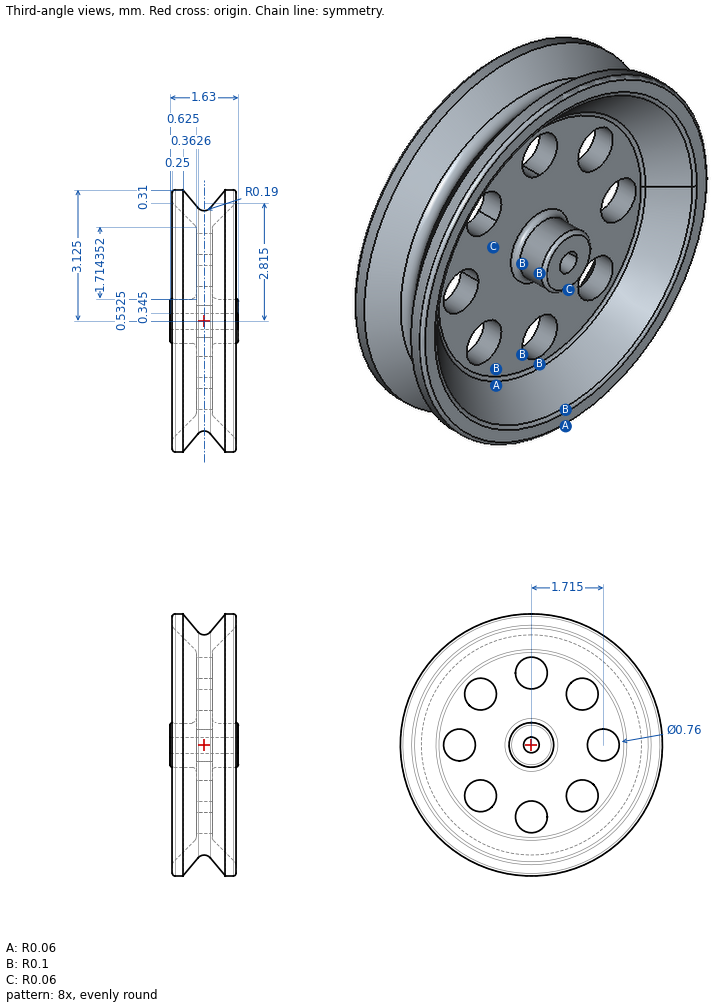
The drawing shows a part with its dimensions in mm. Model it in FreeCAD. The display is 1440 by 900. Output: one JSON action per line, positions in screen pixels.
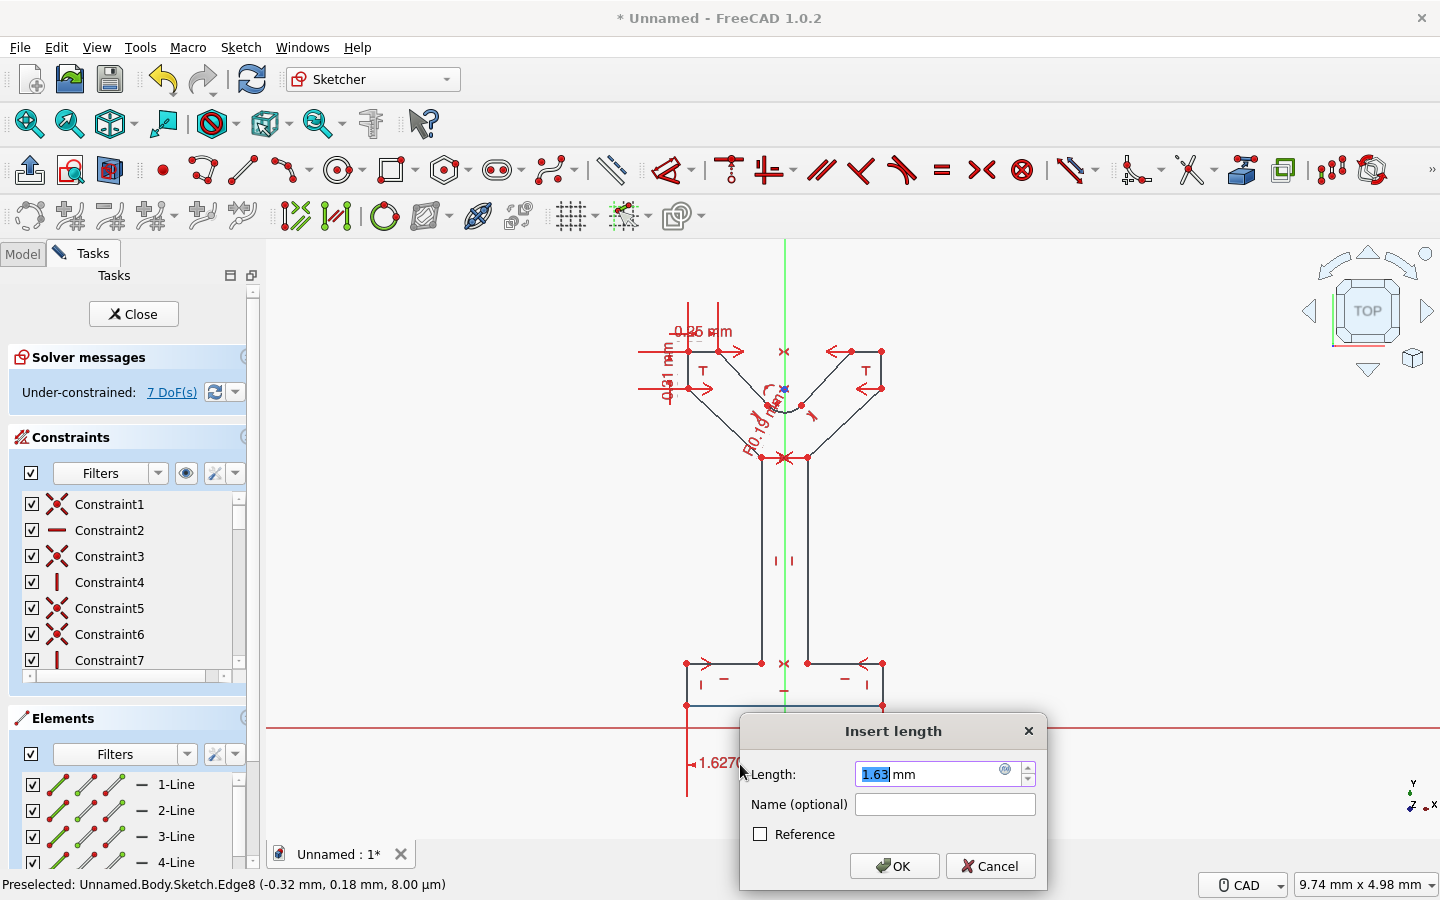
{"action": "type", "text": "1.63"}
{"action": "key", "text": "Return"}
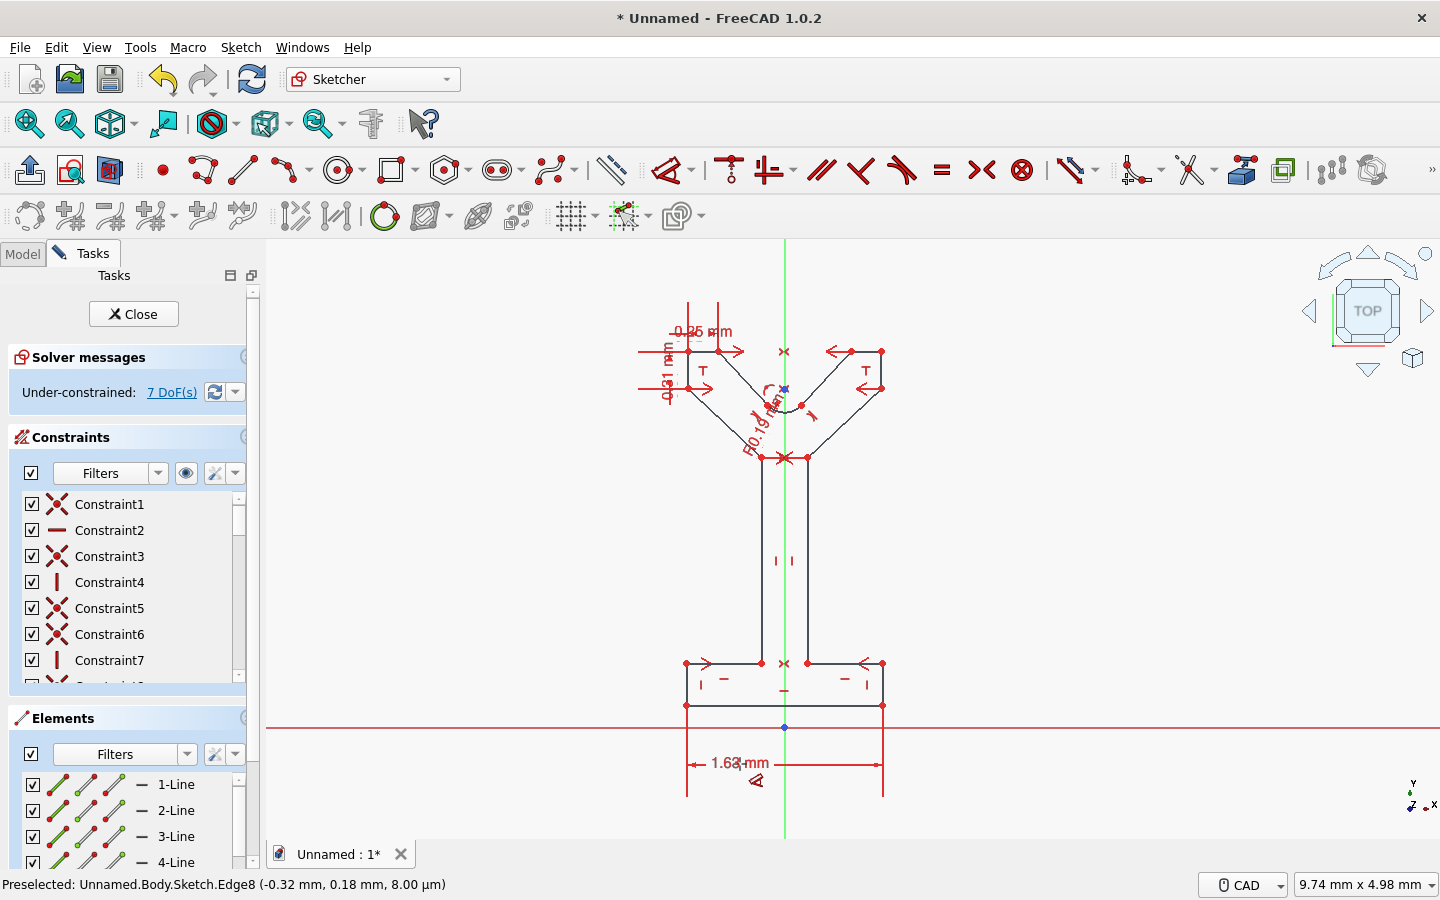
{"action": "left_click", "coordinate": [739, 664]}
{"action": "left_click", "coordinate": [724, 630]}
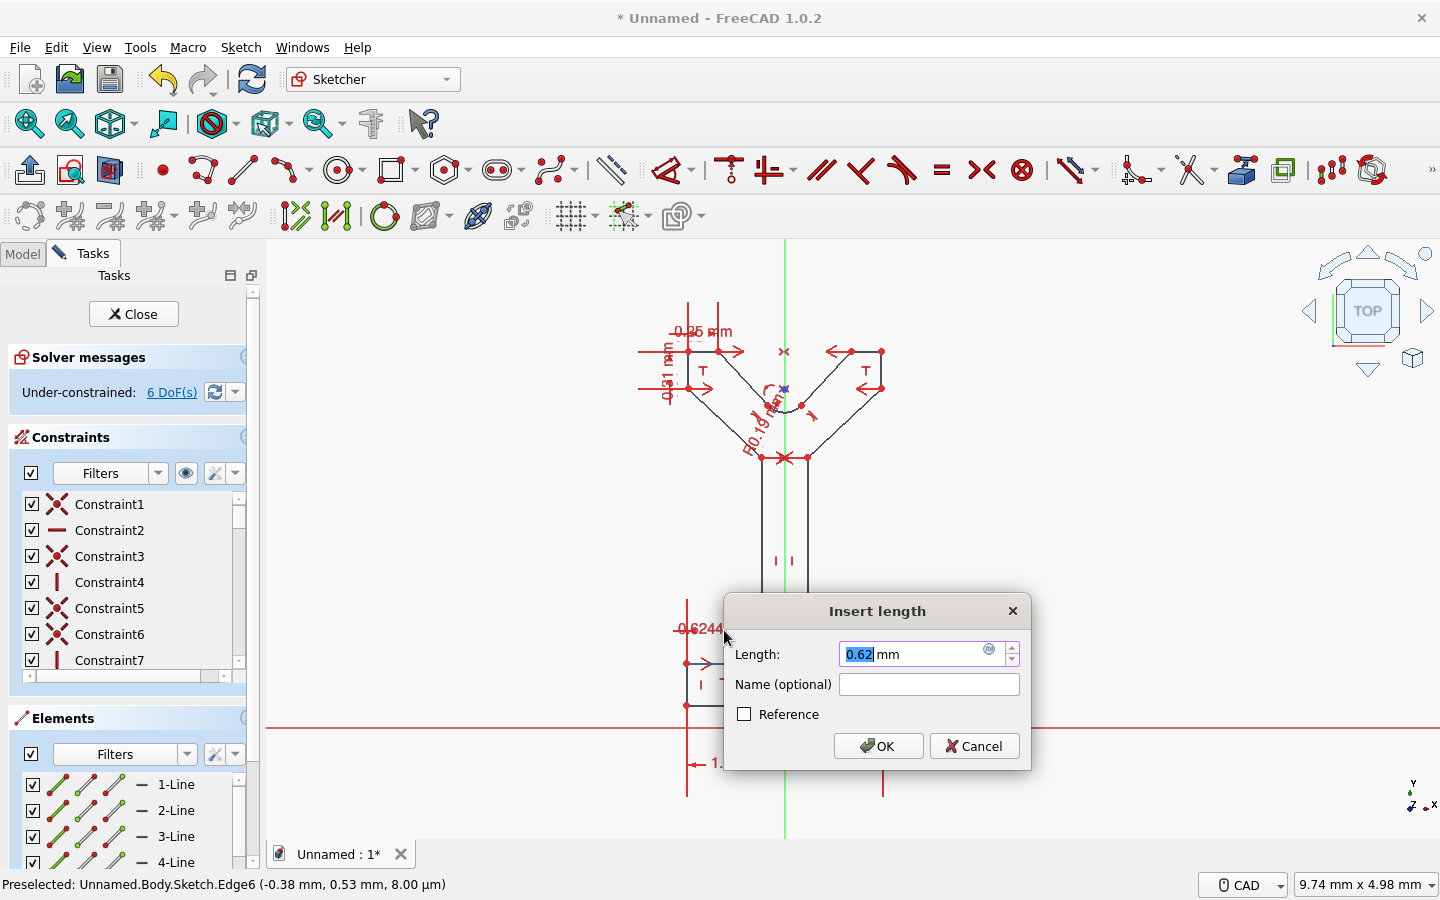
{"action": "type", "text": "0.625"}
{"action": "key", "text": "Return"}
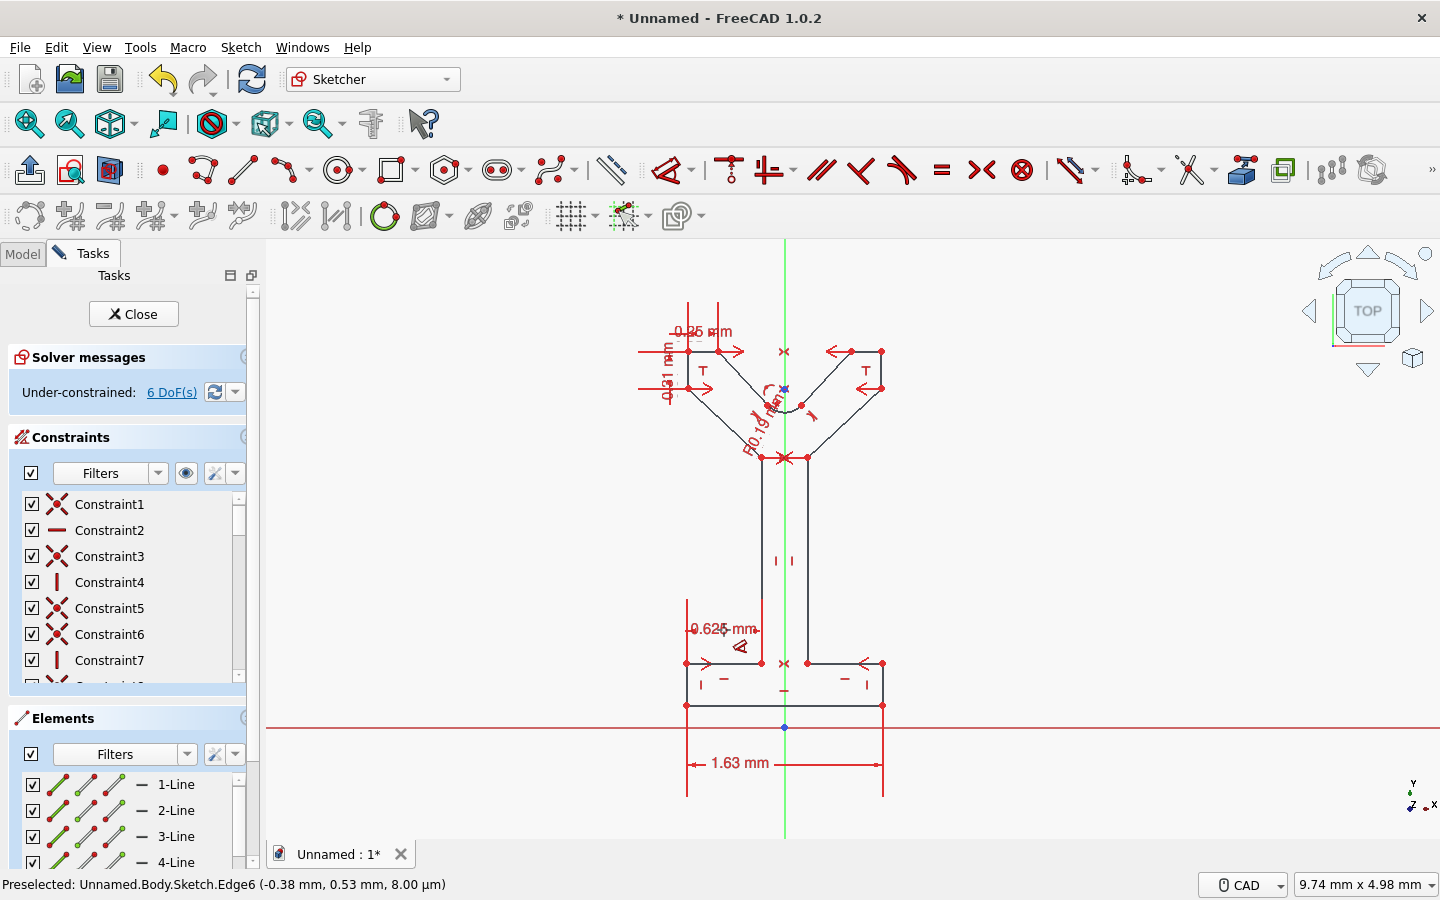
{"action": "left_click", "coordinate": [687, 677]}
{"action": "left_click", "coordinate": [653, 685]}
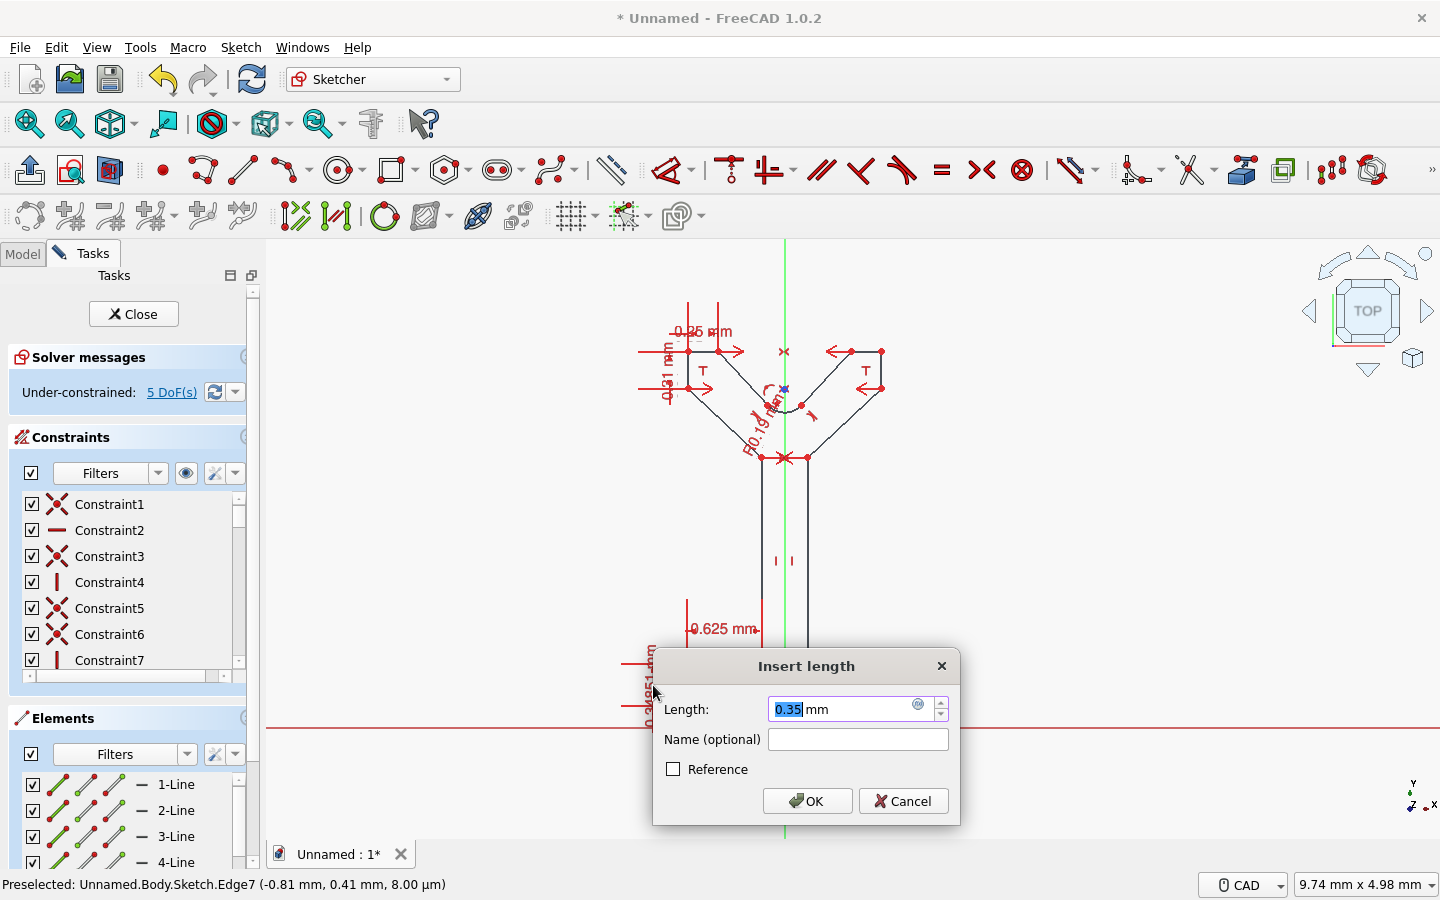
{"action": "type", "text": "0.345"}
{"action": "key", "text": "Return"}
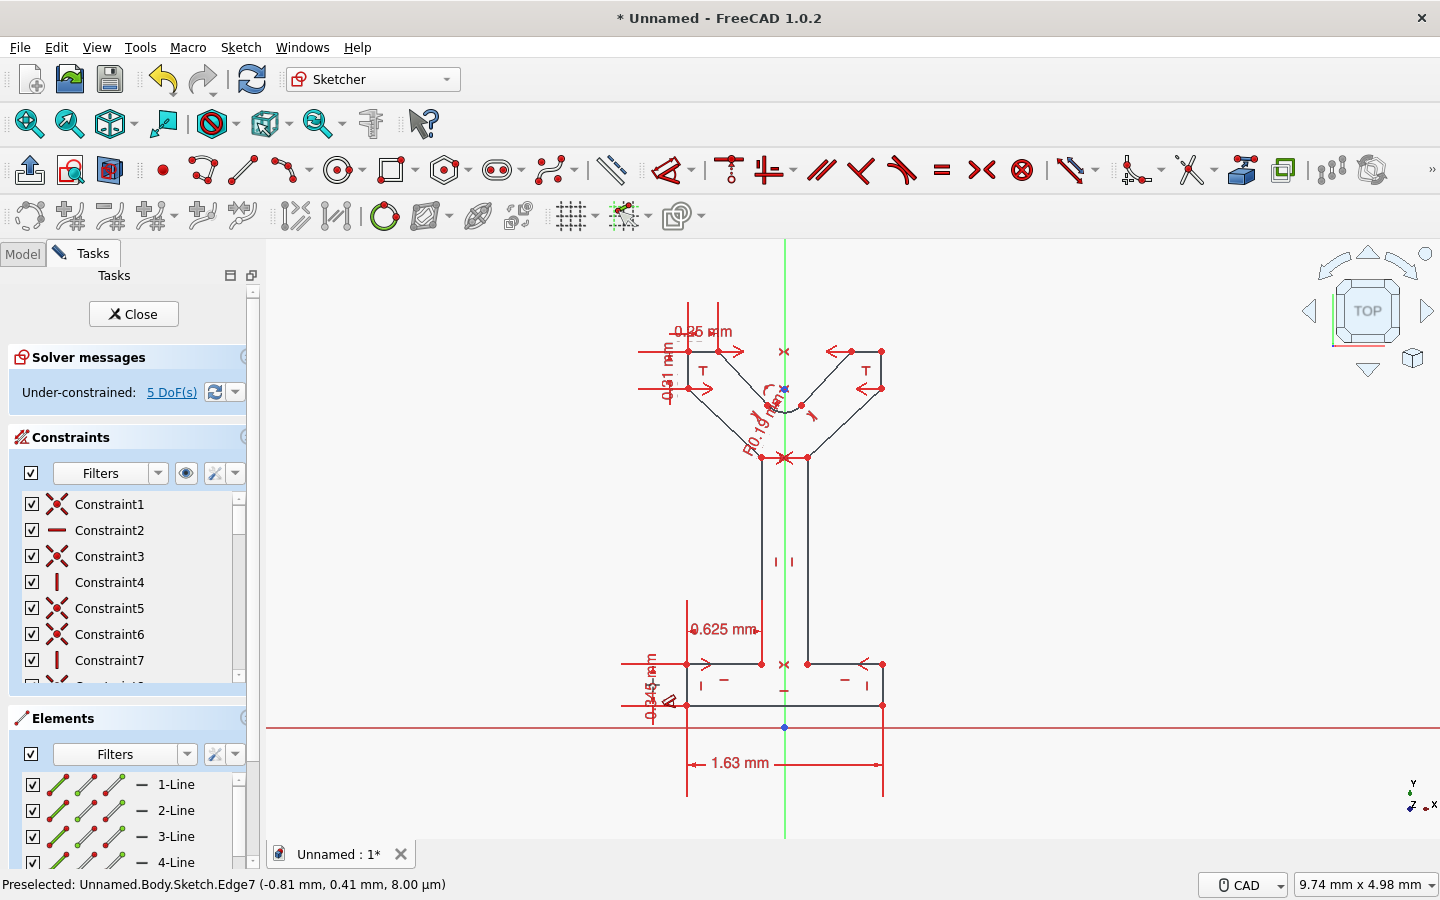
{"action": "left_click", "coordinate": [718, 352]}
{"action": "left_click", "coordinate": [684, 540]}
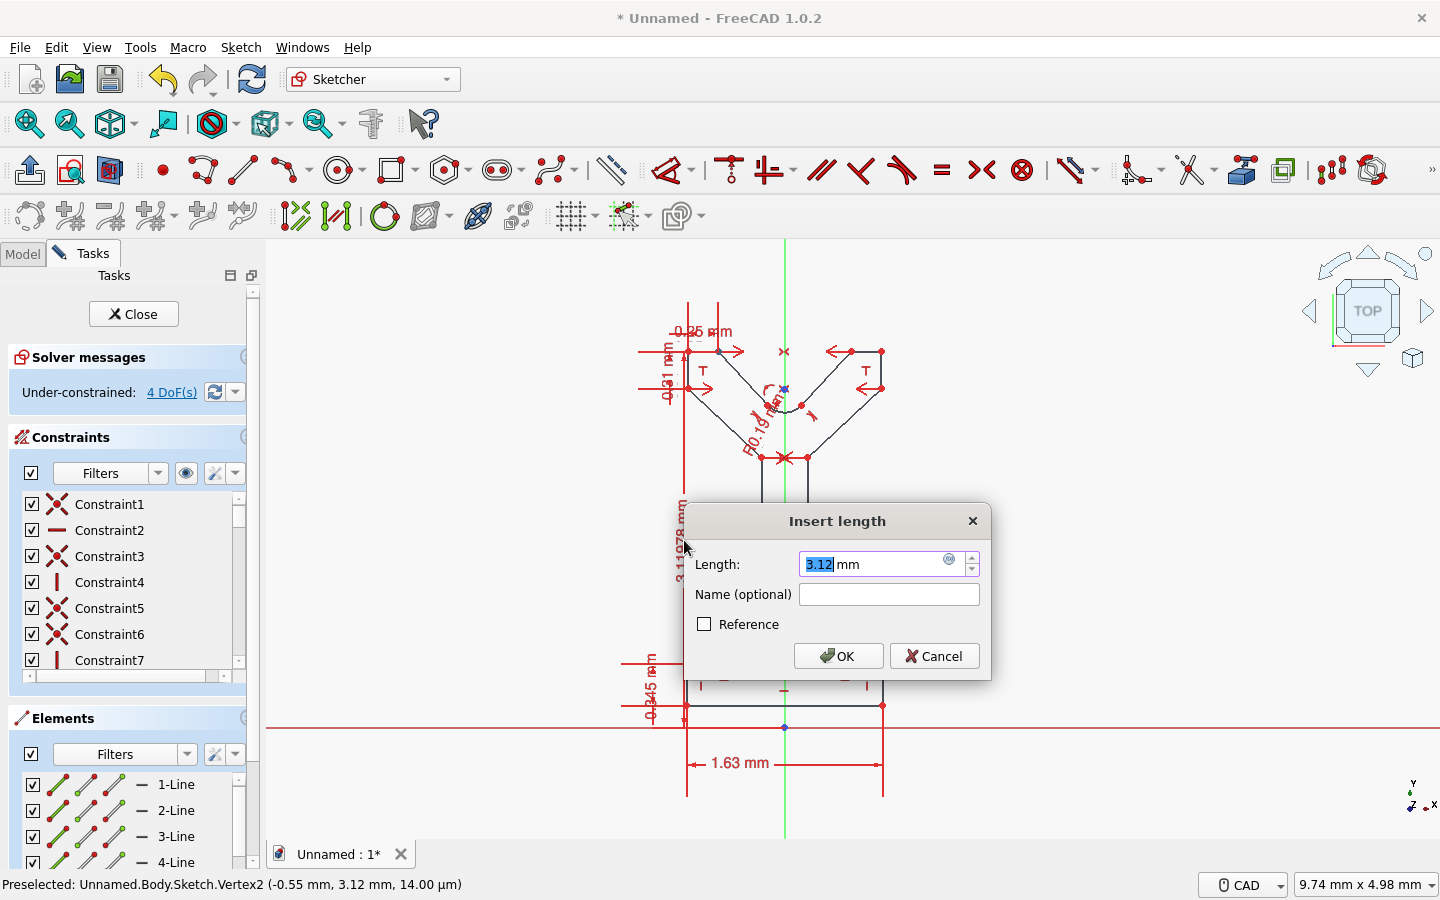
{"action": "type", "text": "3.125"}
{"action": "key", "text": "Return"}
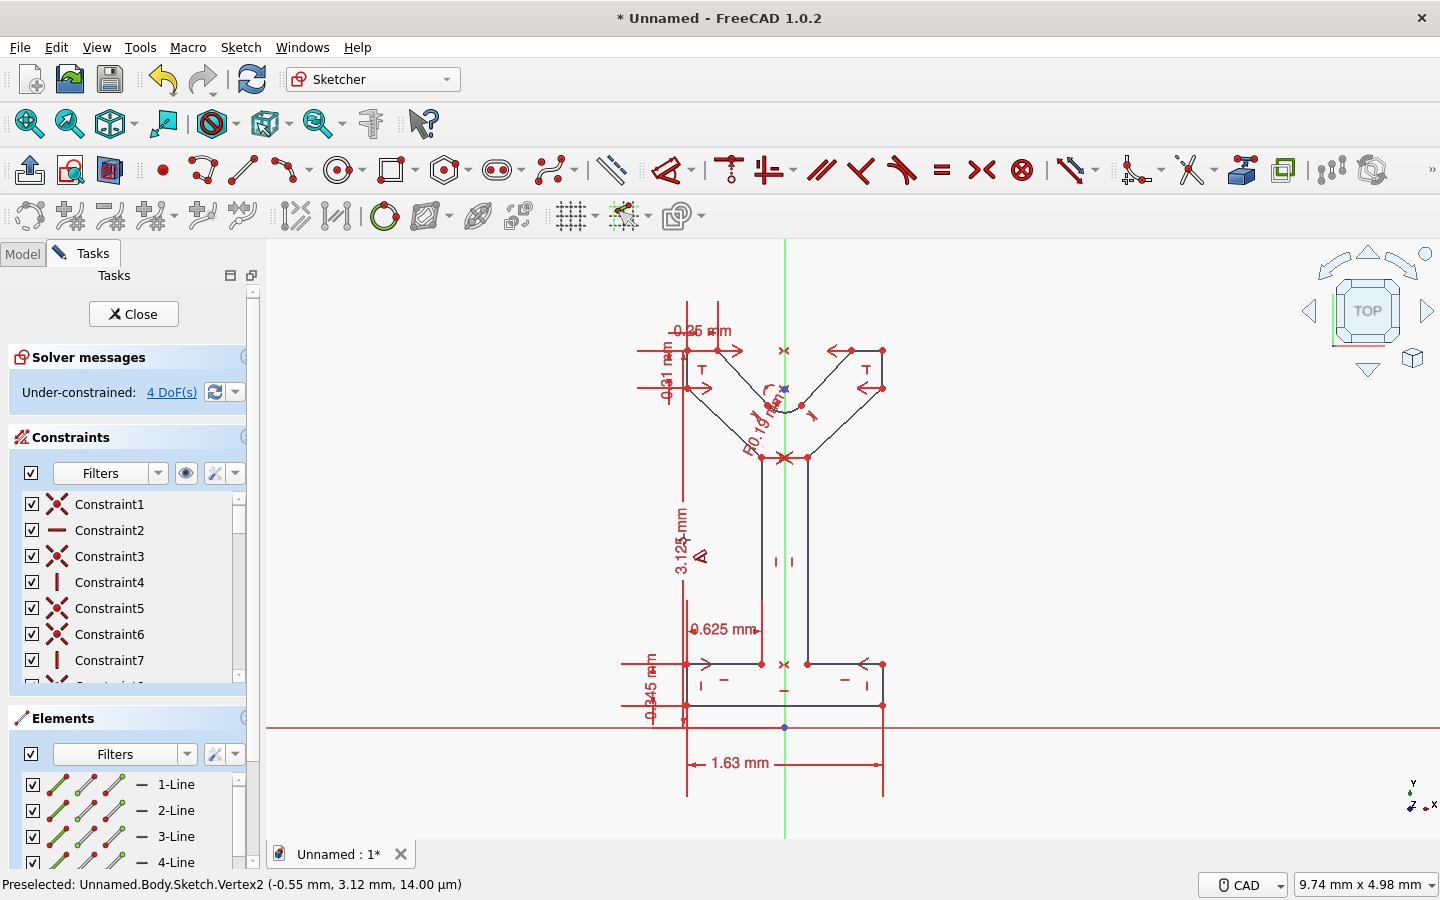
{"action": "left_click", "coordinate": [785, 390]}
{"action": "left_click", "coordinate": [843, 559]}